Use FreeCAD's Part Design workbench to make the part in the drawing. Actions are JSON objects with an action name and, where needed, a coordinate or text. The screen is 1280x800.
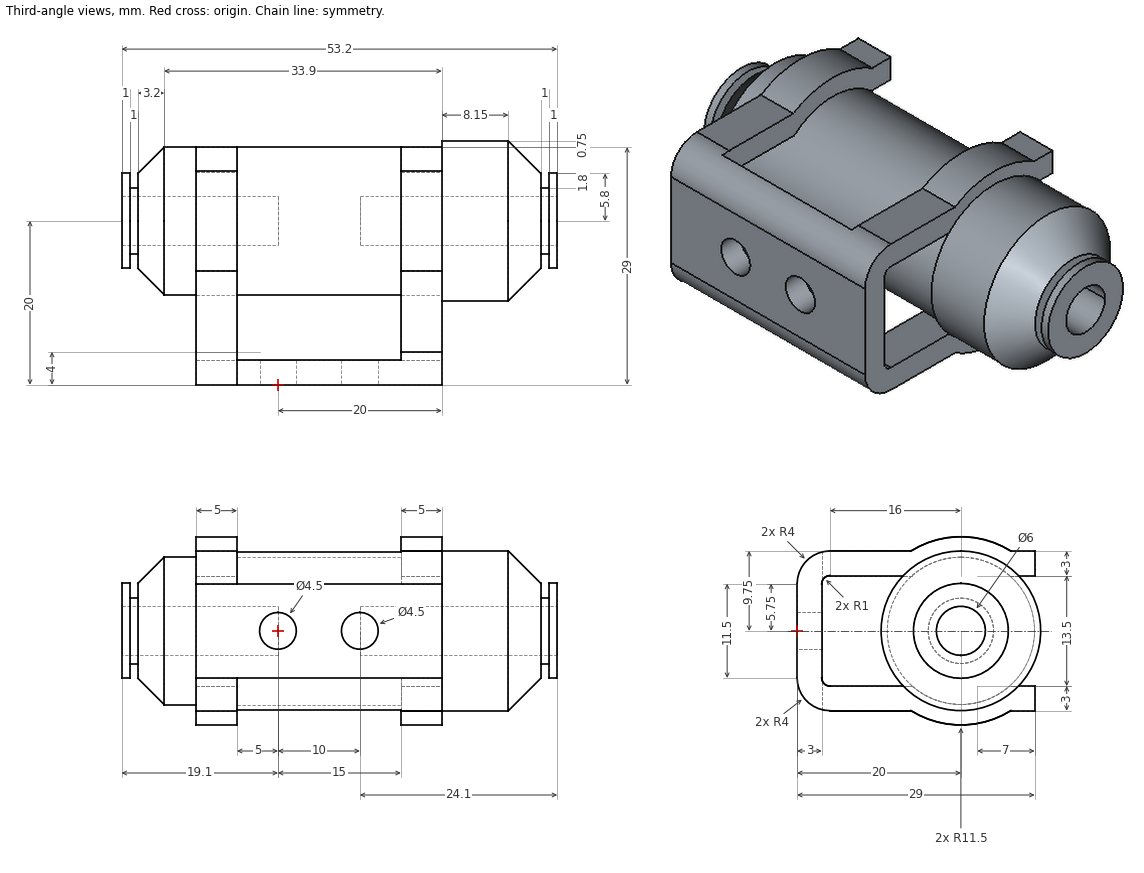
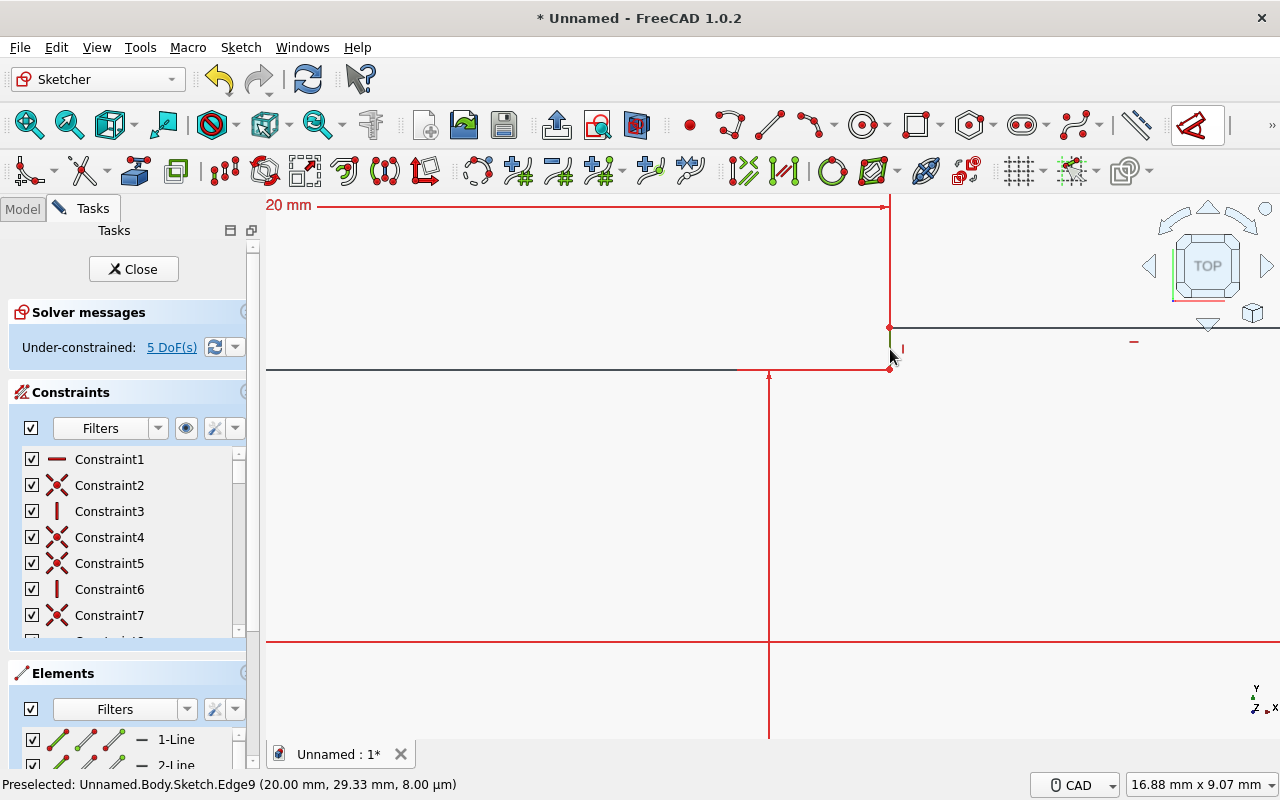
{"action": "left_click", "coordinate": [1218, 126]}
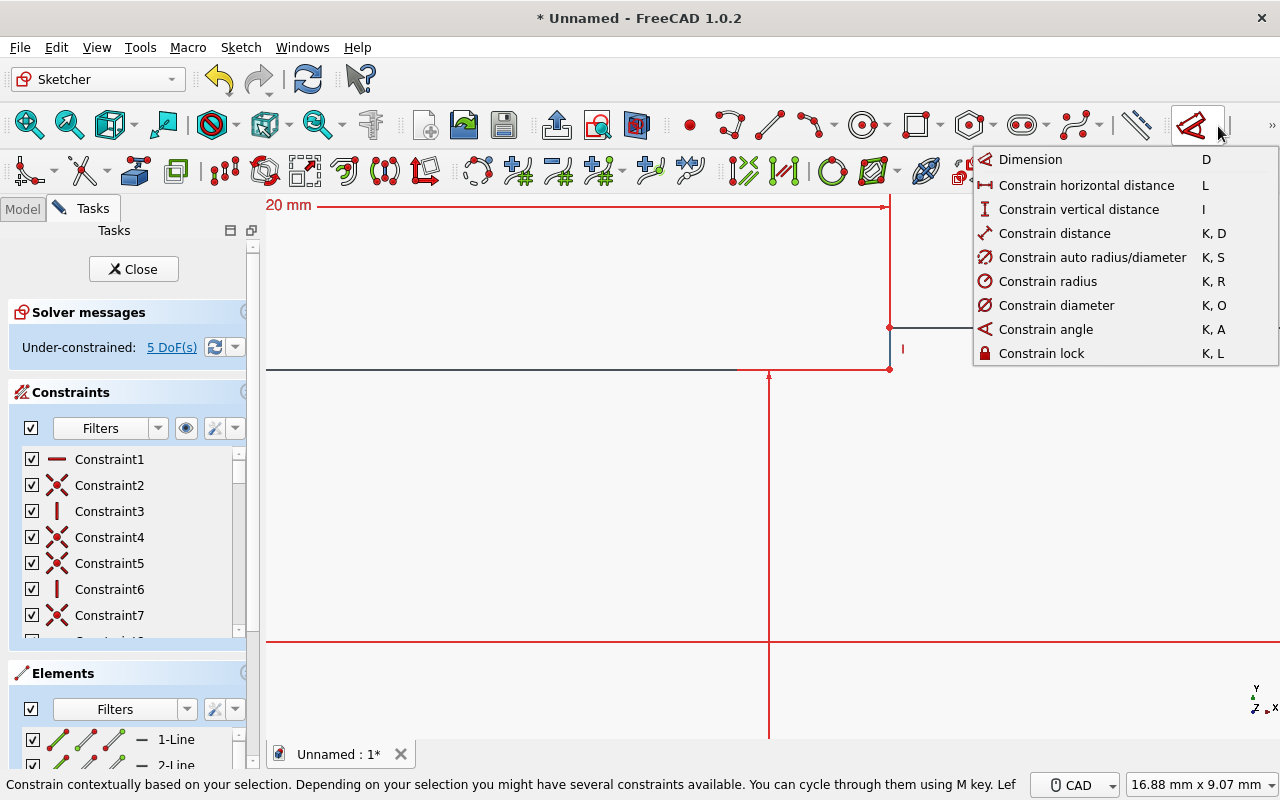
{"action": "left_click", "coordinate": [1126, 209]}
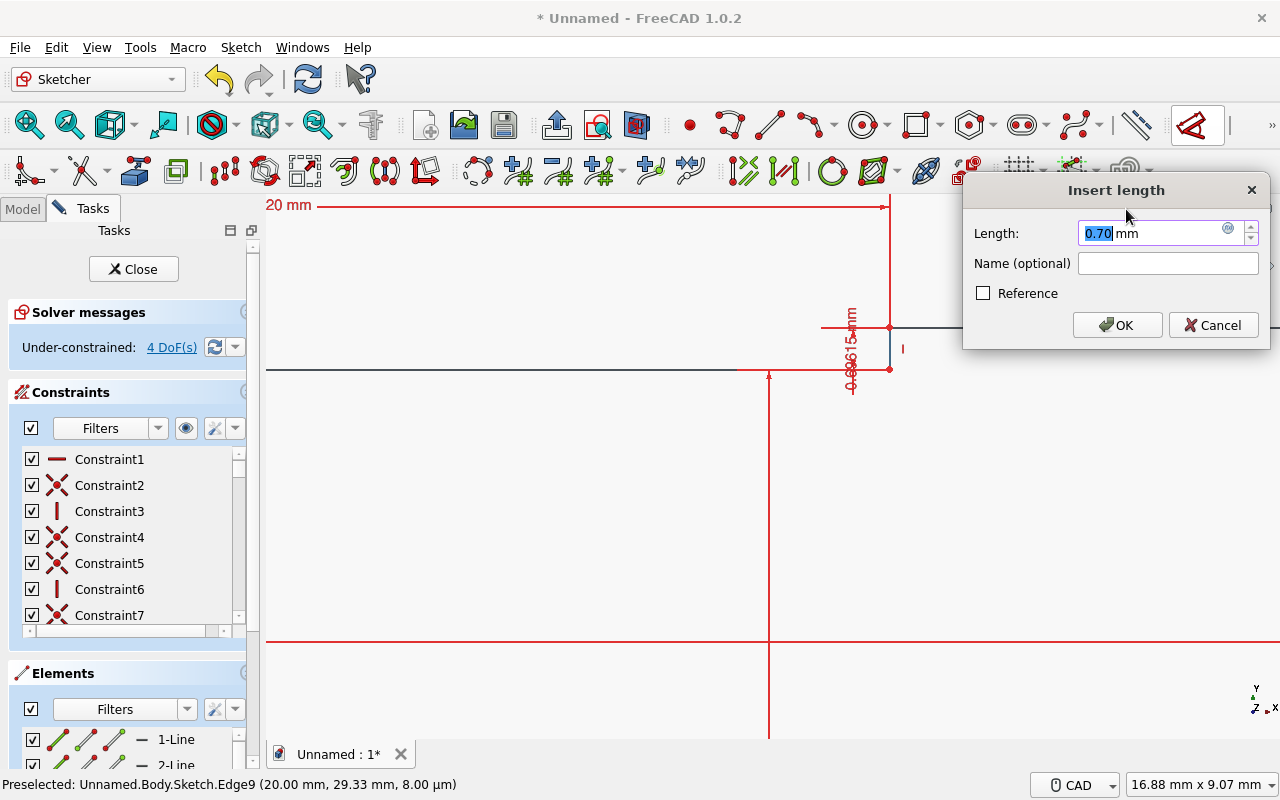
{"action": "type", "text": "0.75"}
{"action": "key", "text": "Return"}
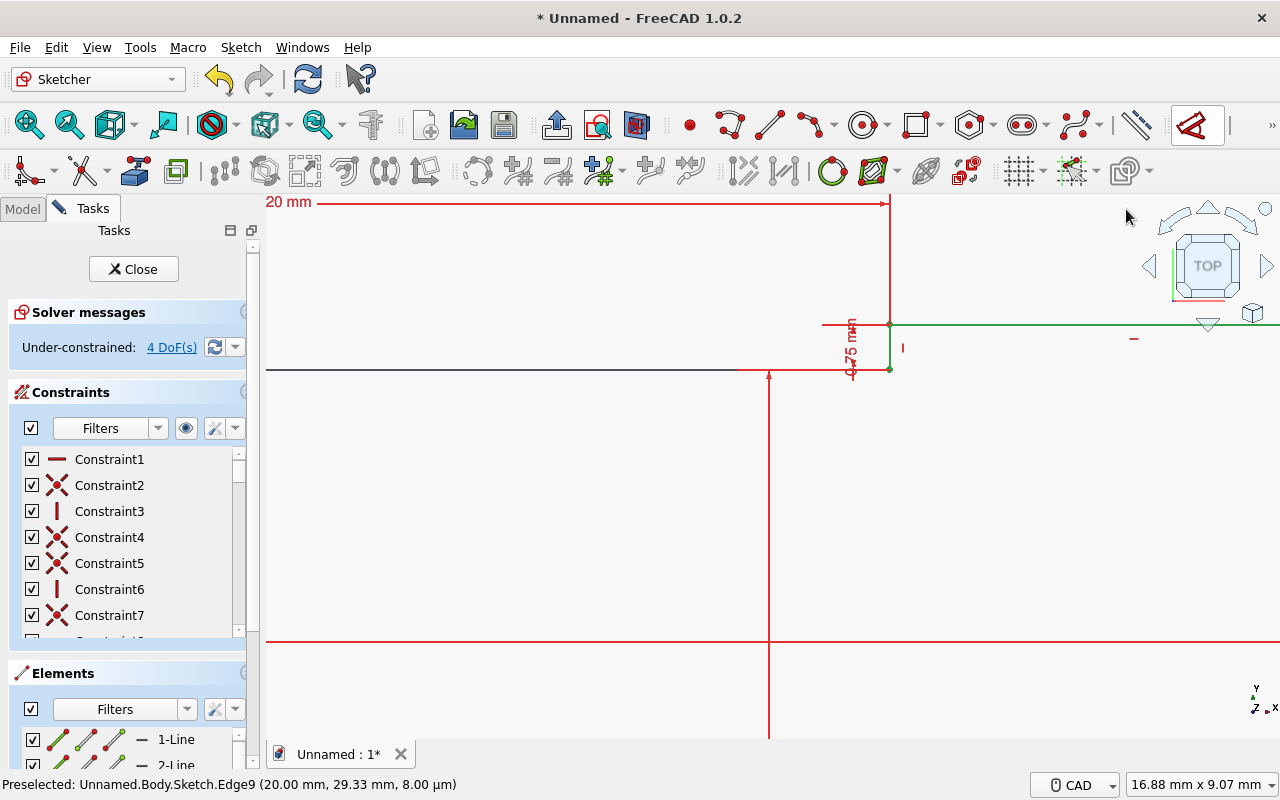
{"action": "scroll", "coordinate": [893, 349], "scroll_direction": "down", "scroll_amount": 10}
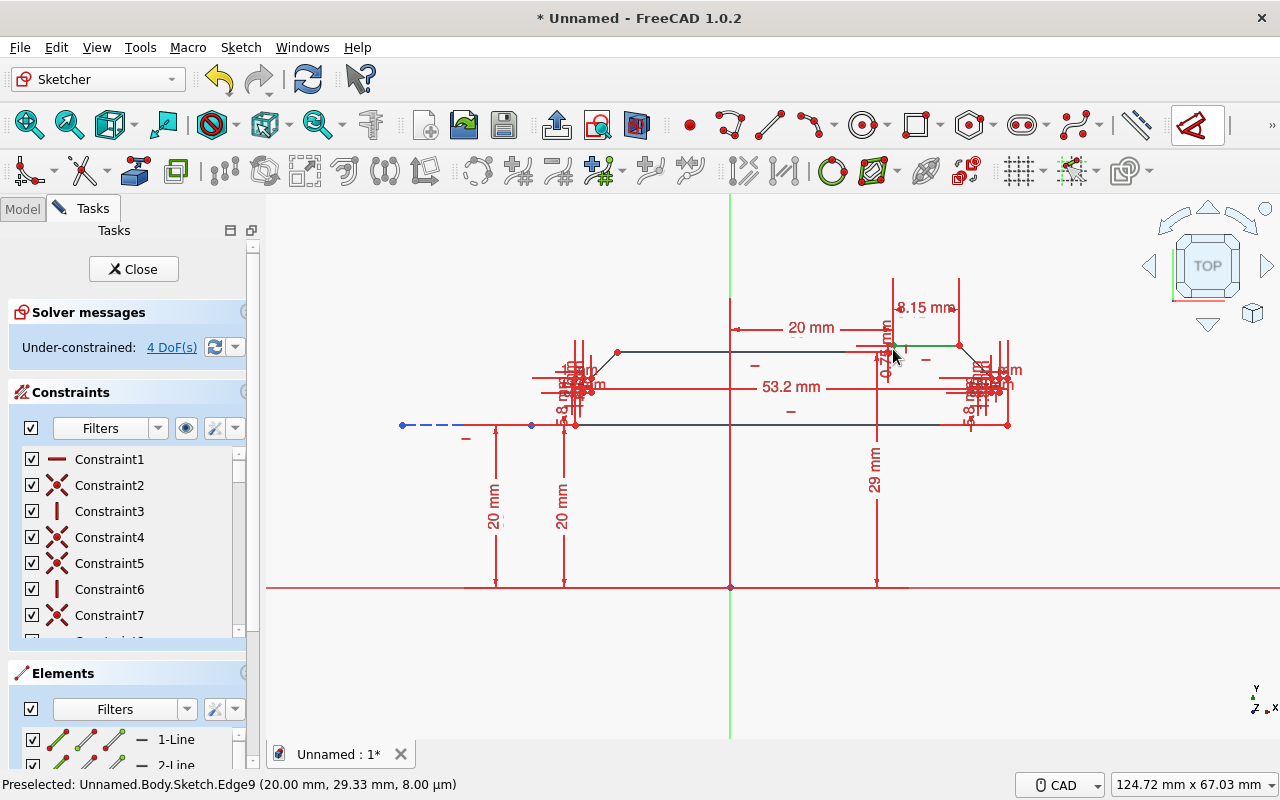
{"action": "left_click", "coordinate": [838, 352]}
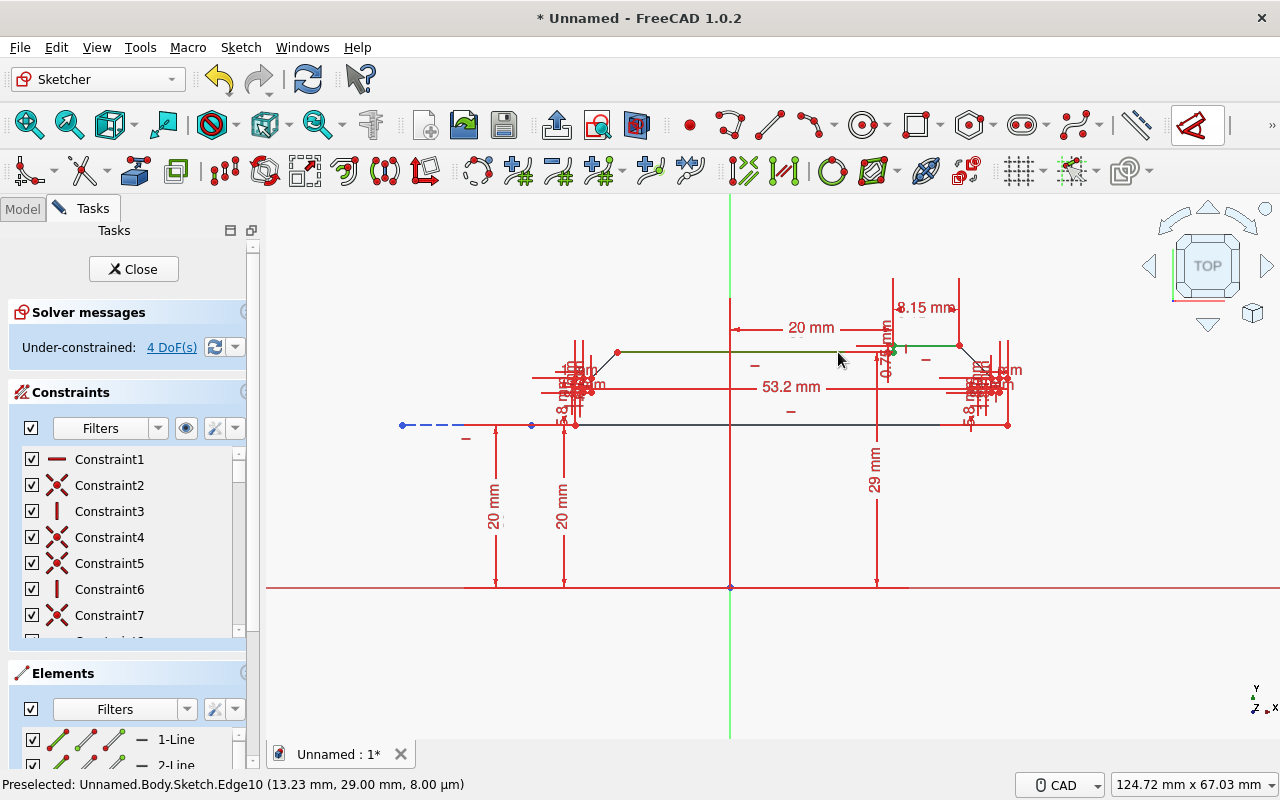
{"action": "left_click", "coordinate": [1218, 126]}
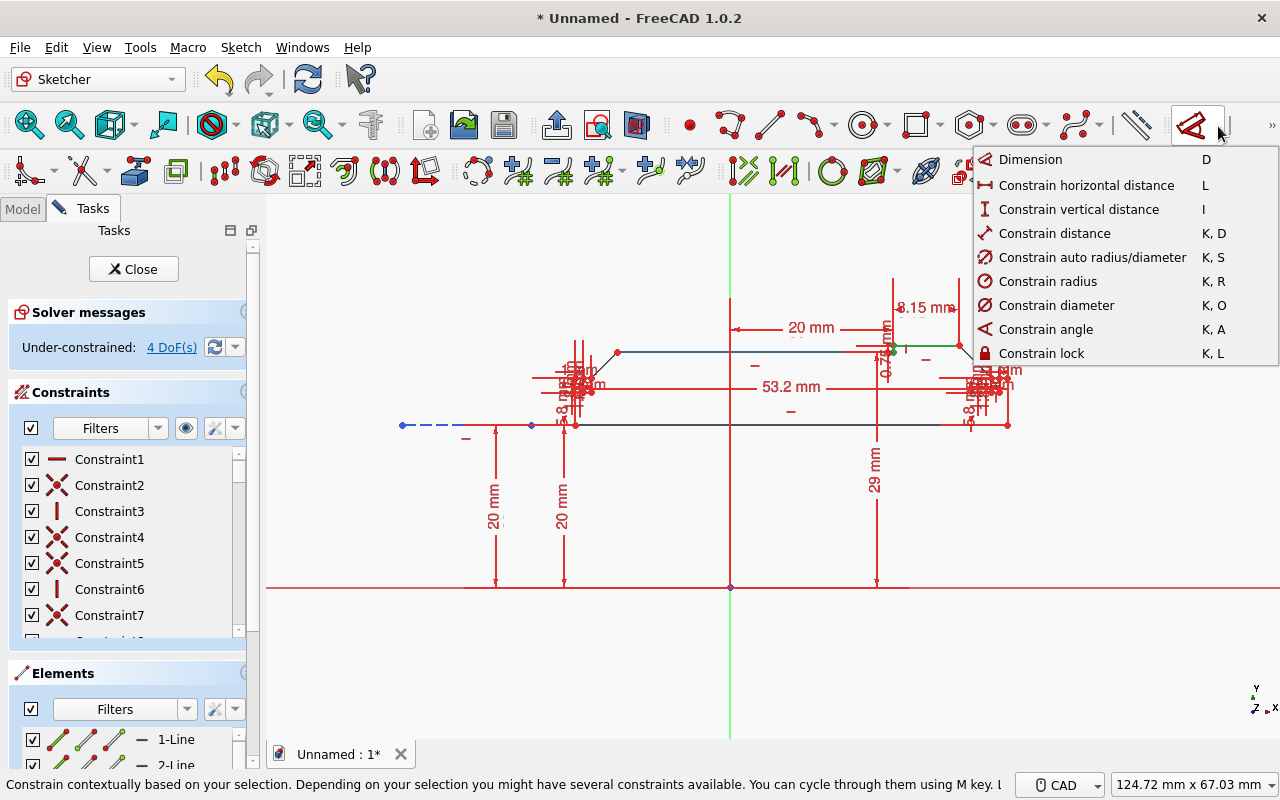
{"action": "left_click", "coordinate": [1126, 185]}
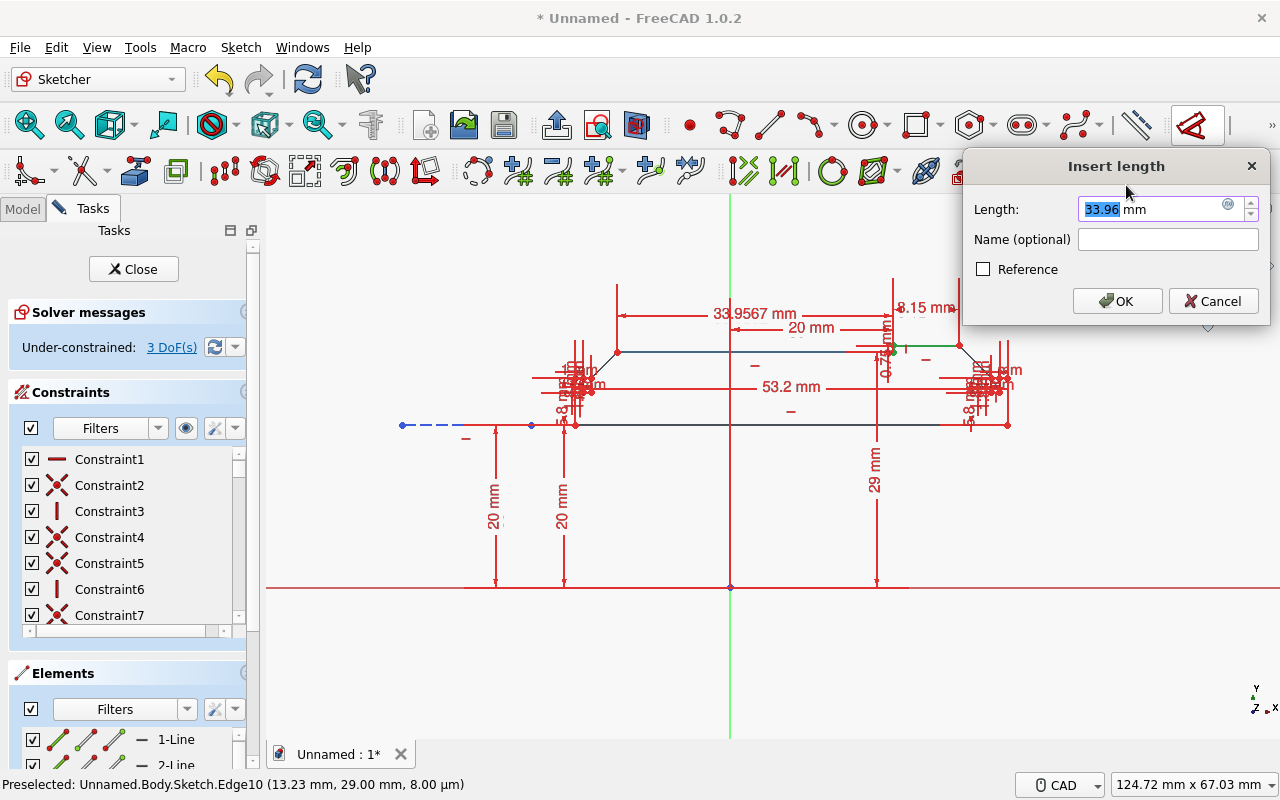
{"action": "type", "text": "33.9"}
{"action": "key", "text": "Return"}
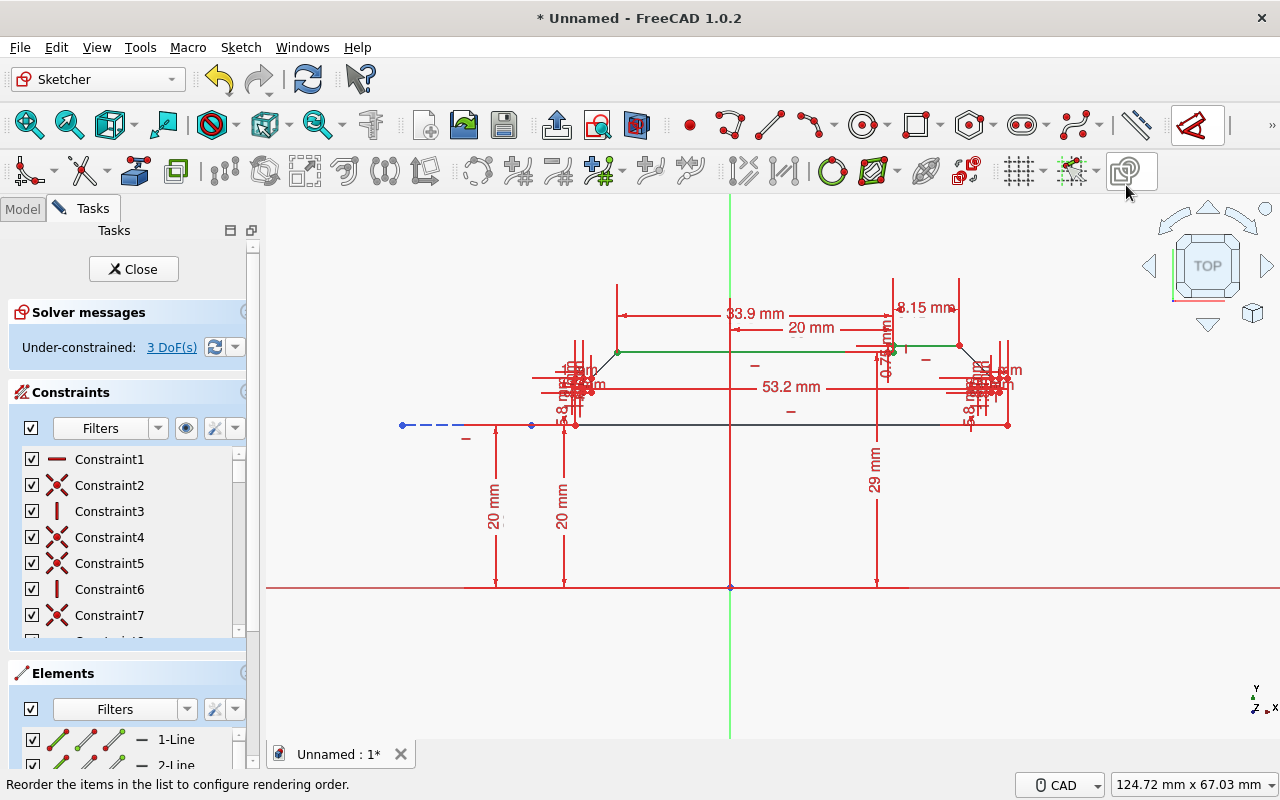
{"action": "scroll", "coordinate": [610, 360], "scroll_direction": "up", "scroll_amount": 3}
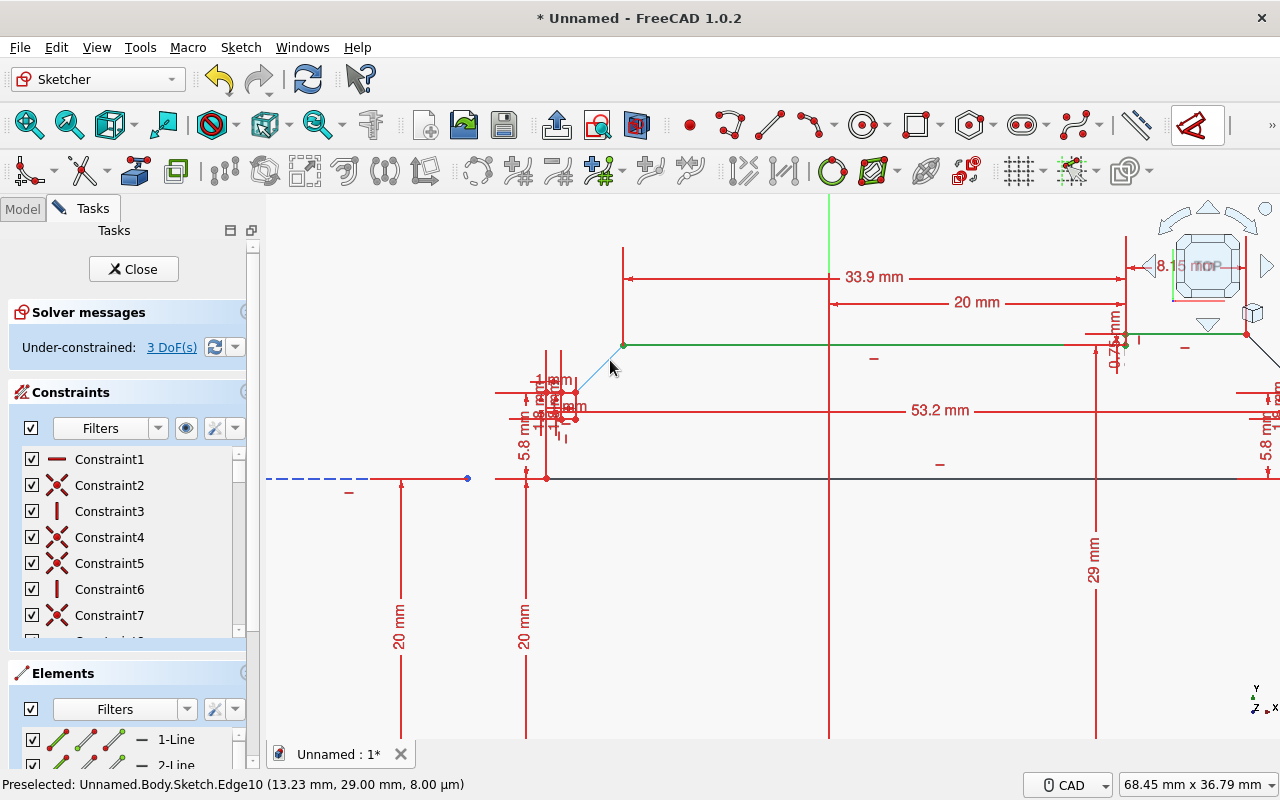
{"action": "left_click", "coordinate": [609, 359]}